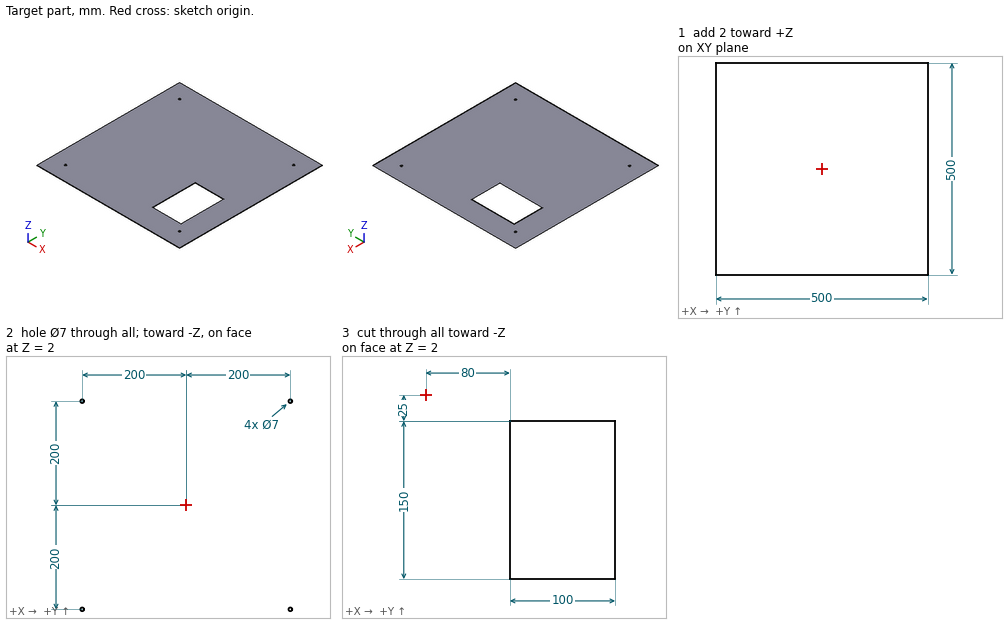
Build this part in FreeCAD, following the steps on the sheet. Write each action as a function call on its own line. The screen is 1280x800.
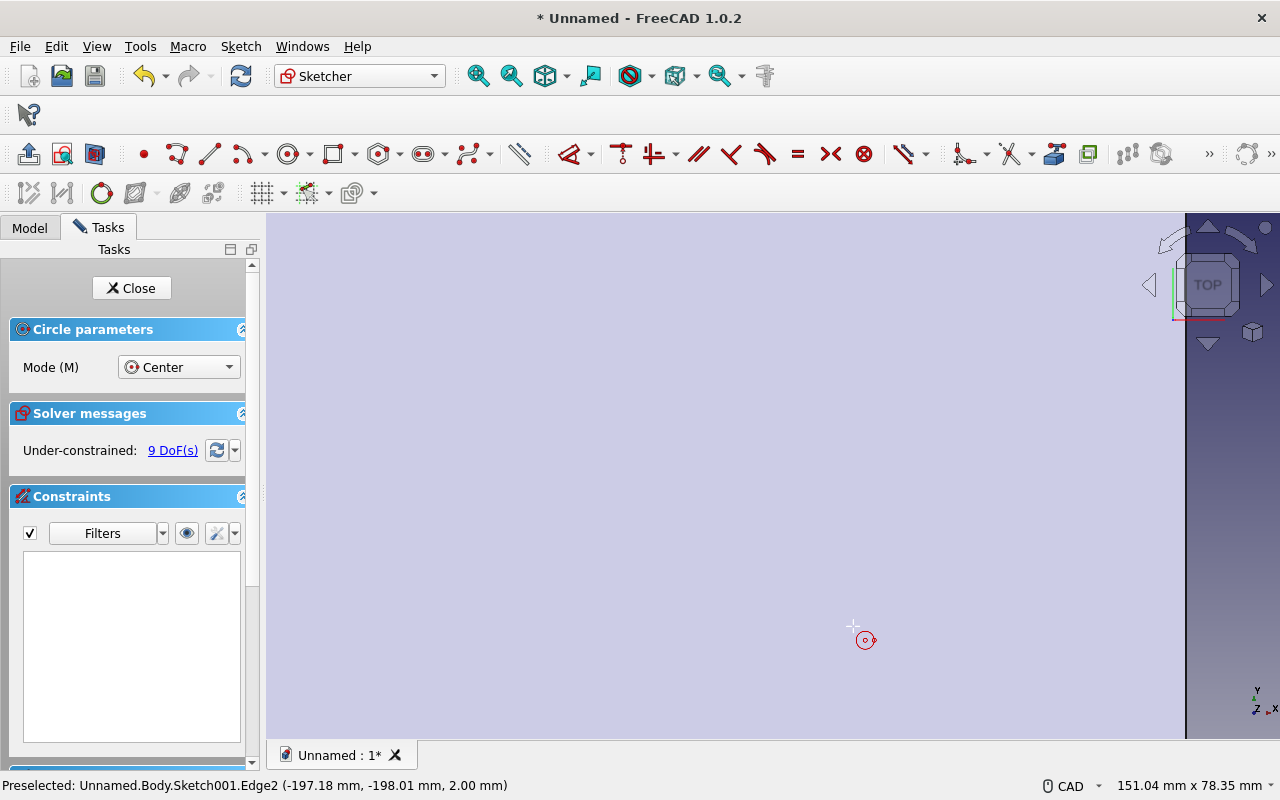
scroll(854, 626, down, 11)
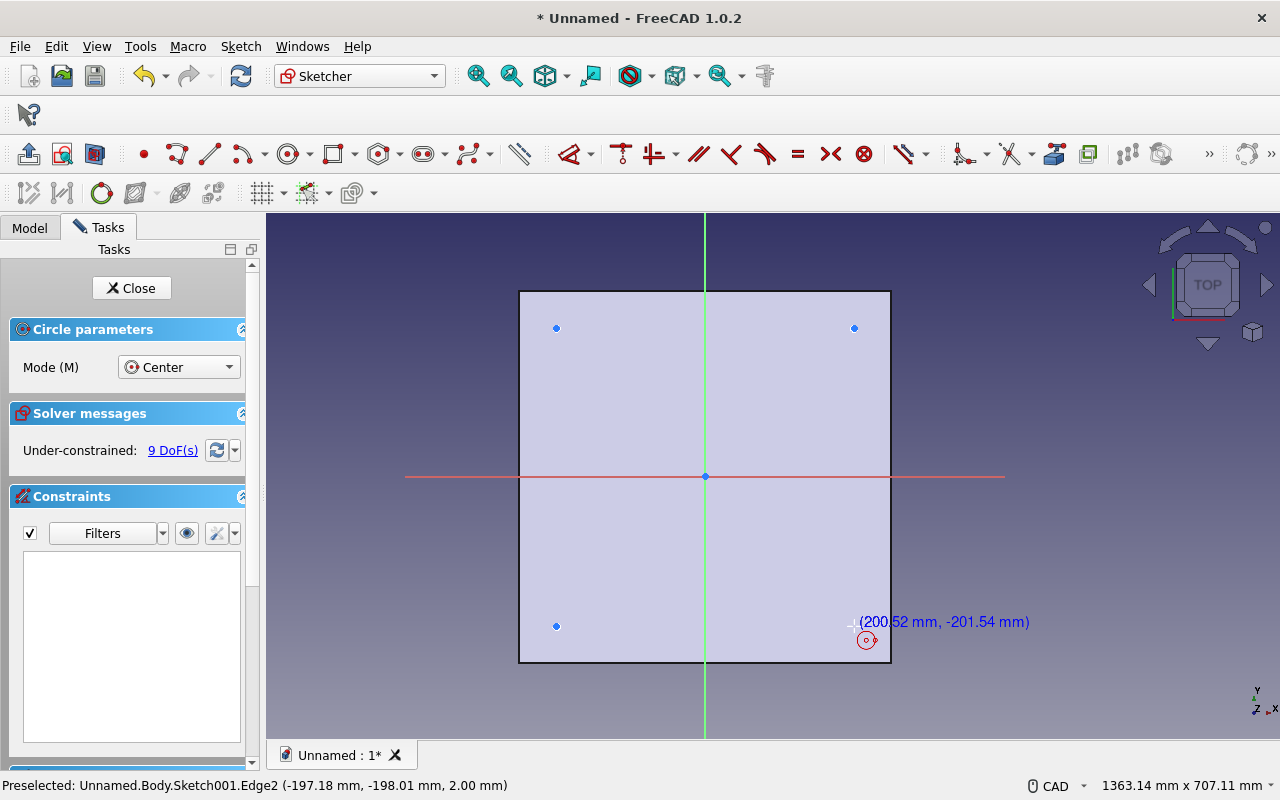
click(854, 626)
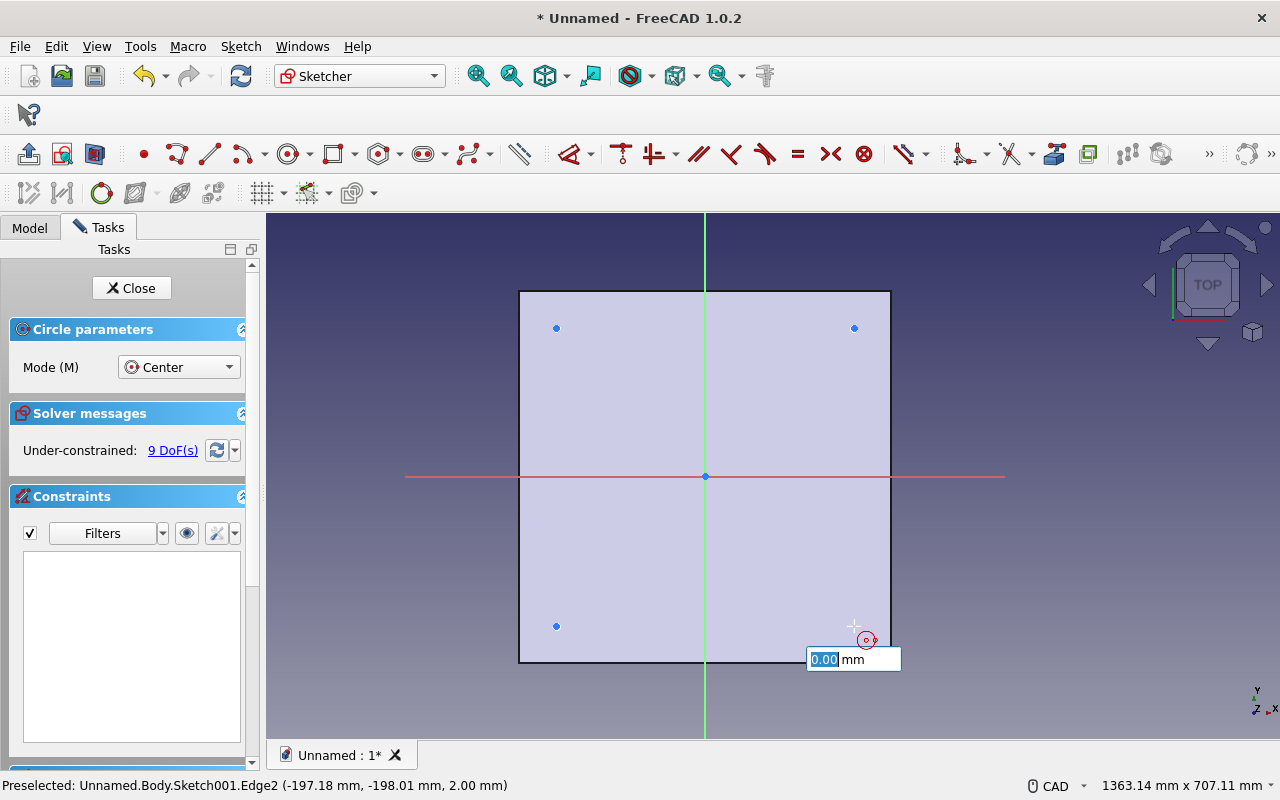
scroll(856, 624, up, 10)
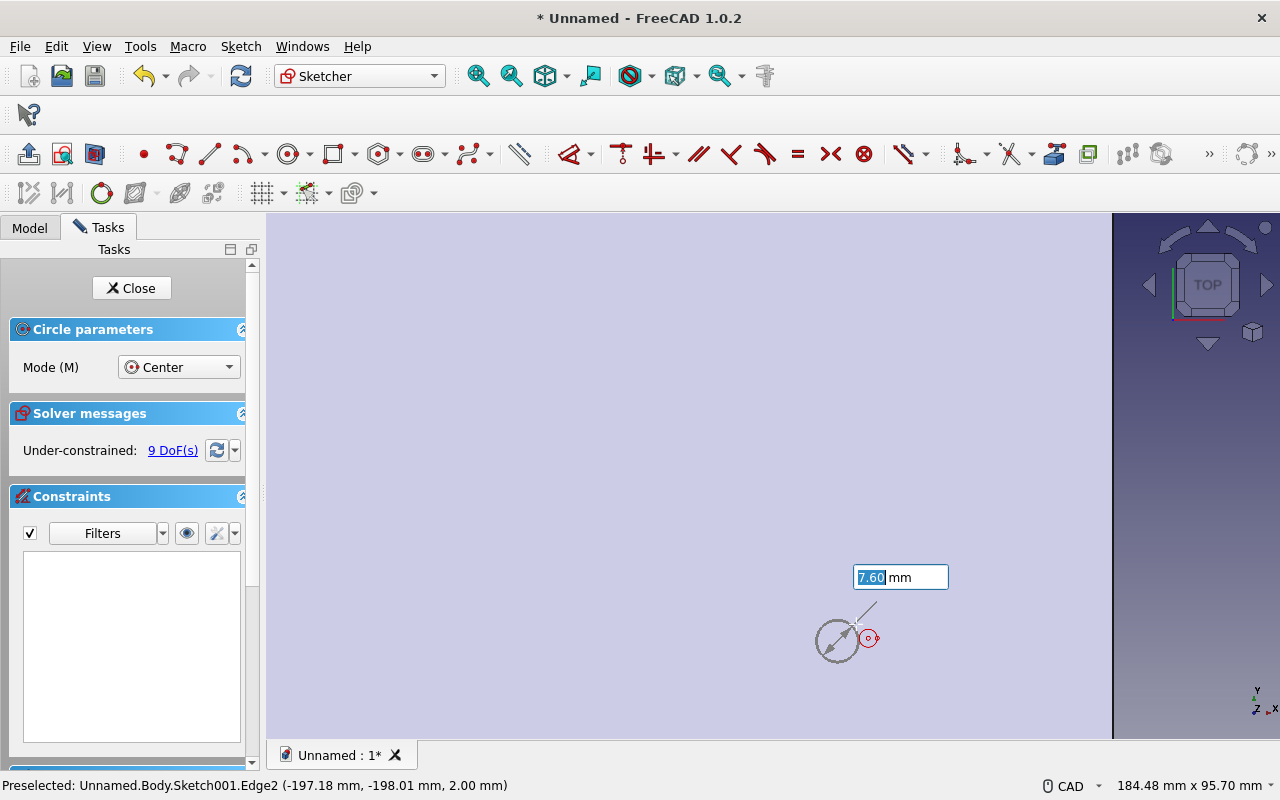
click(852, 618)
key(Escape)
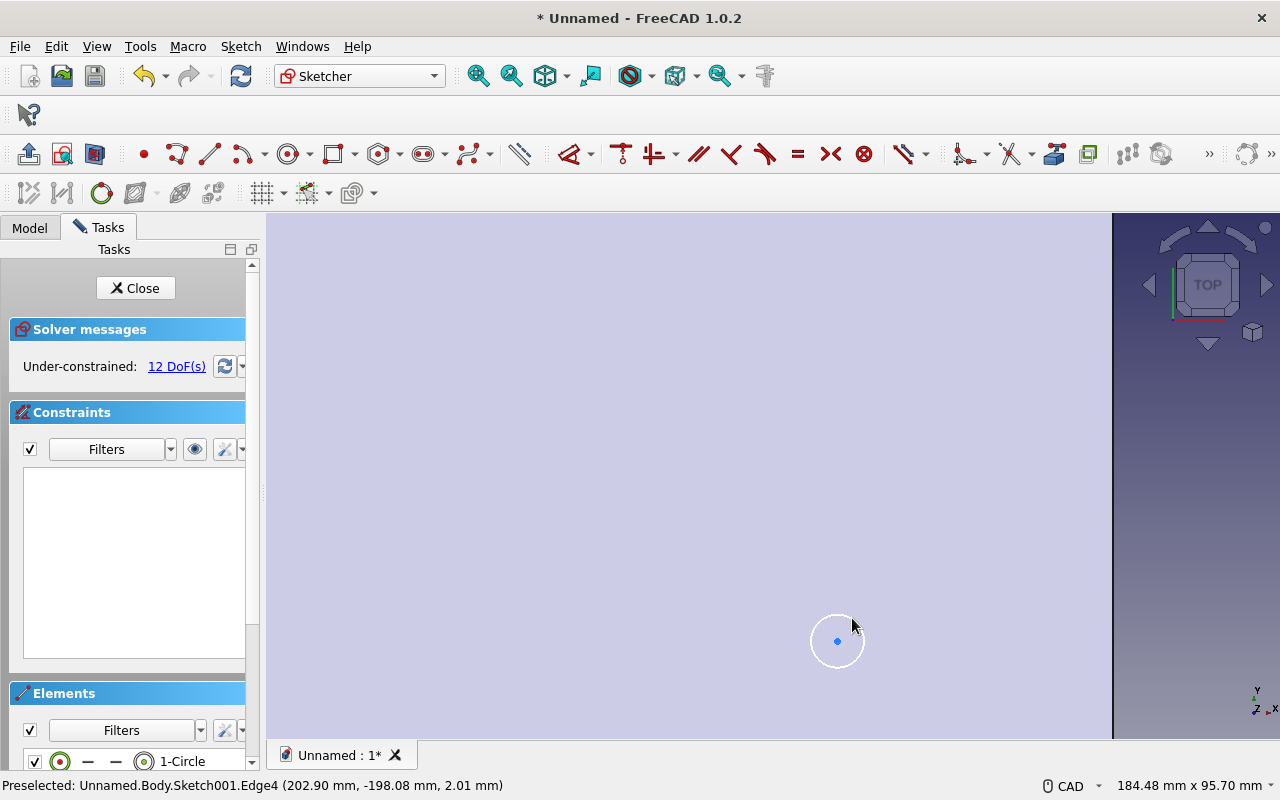
scroll(856, 624, down, 10)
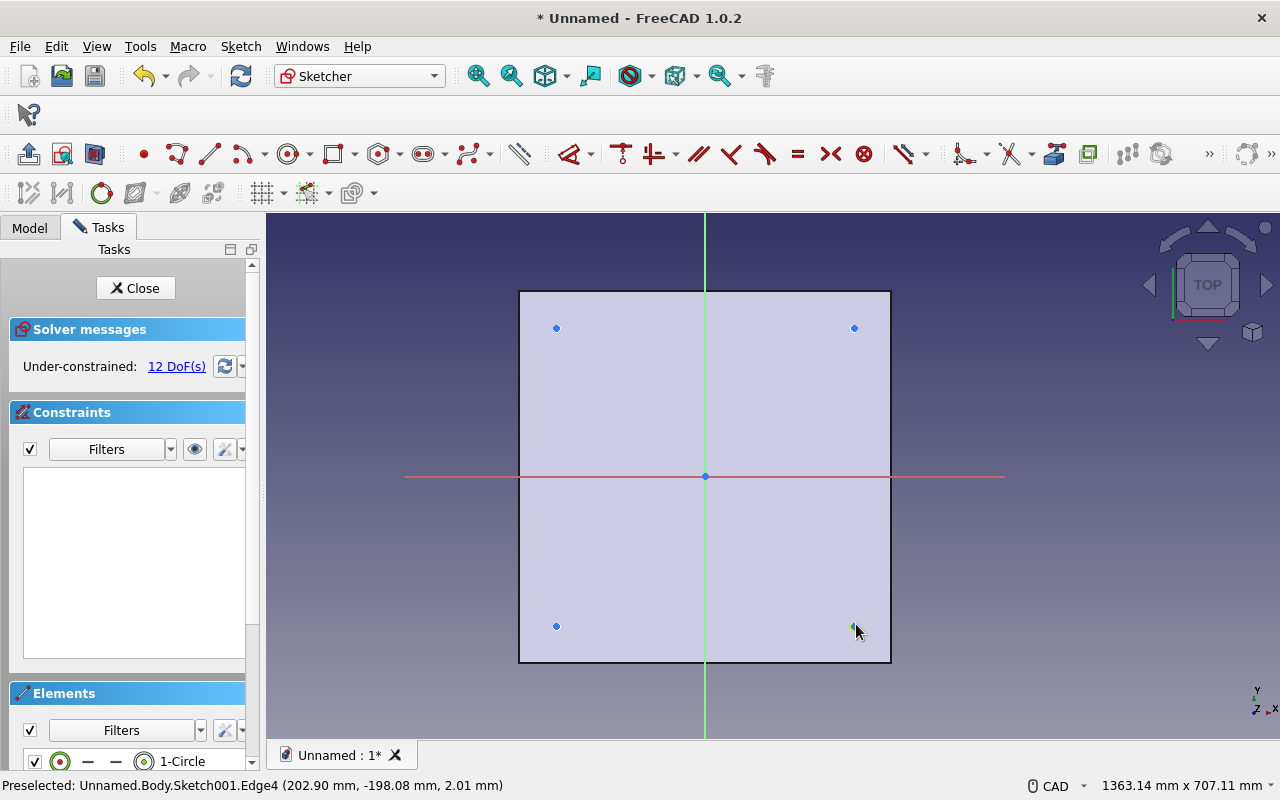
scroll(559, 327, up, 8)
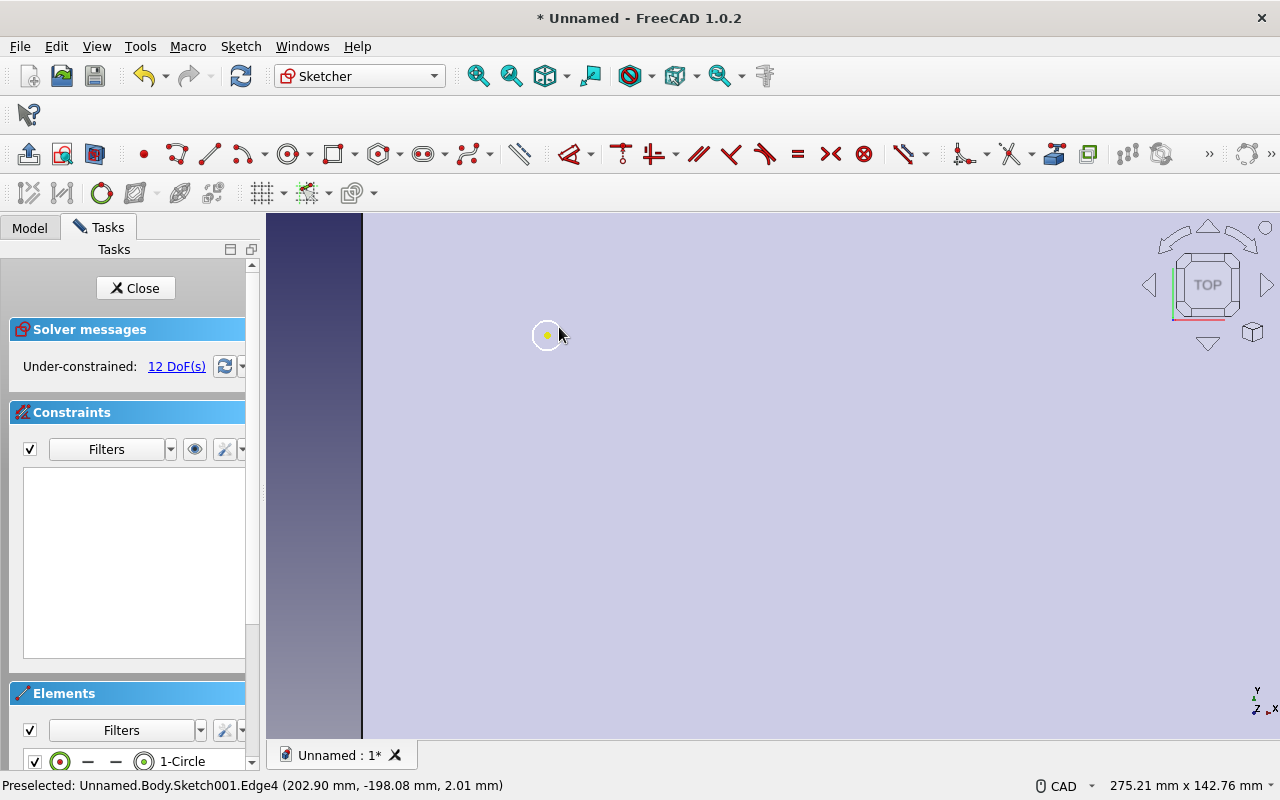
click(558, 325)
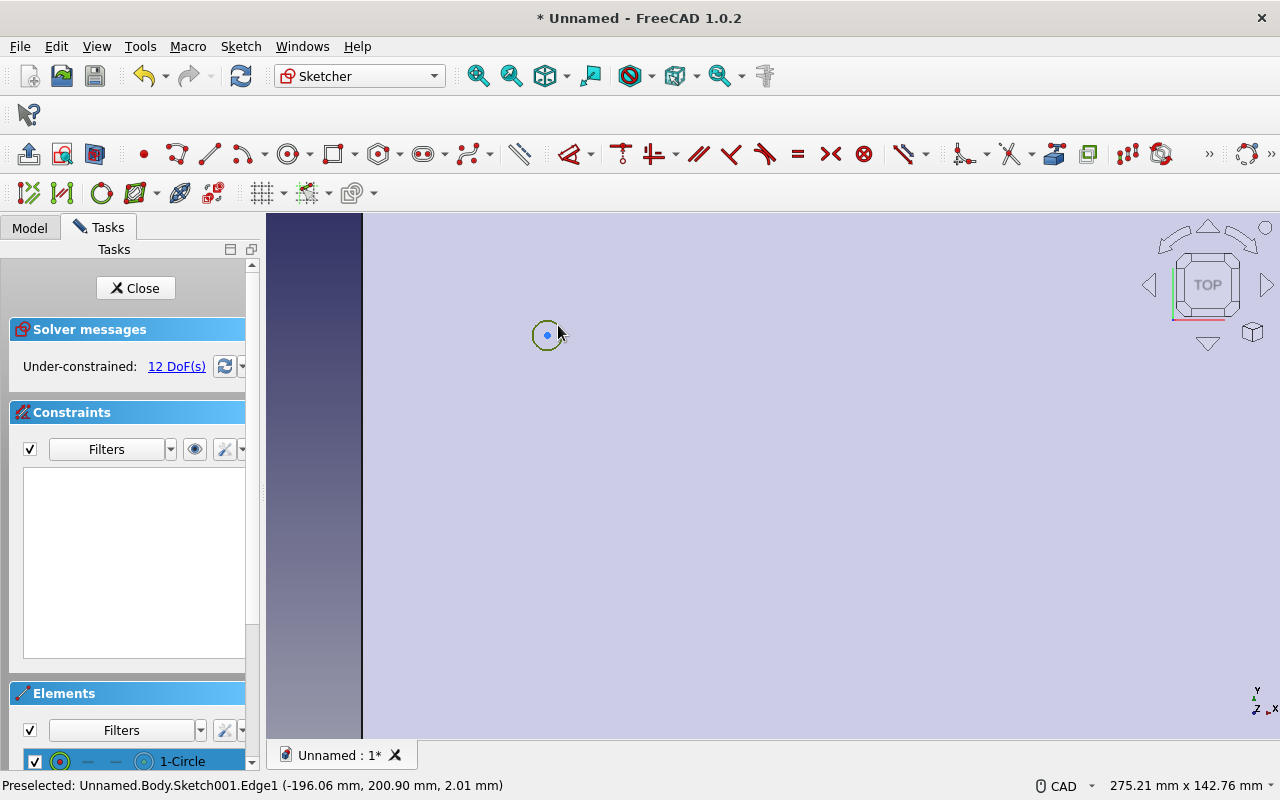
scroll(558, 326, down, 8)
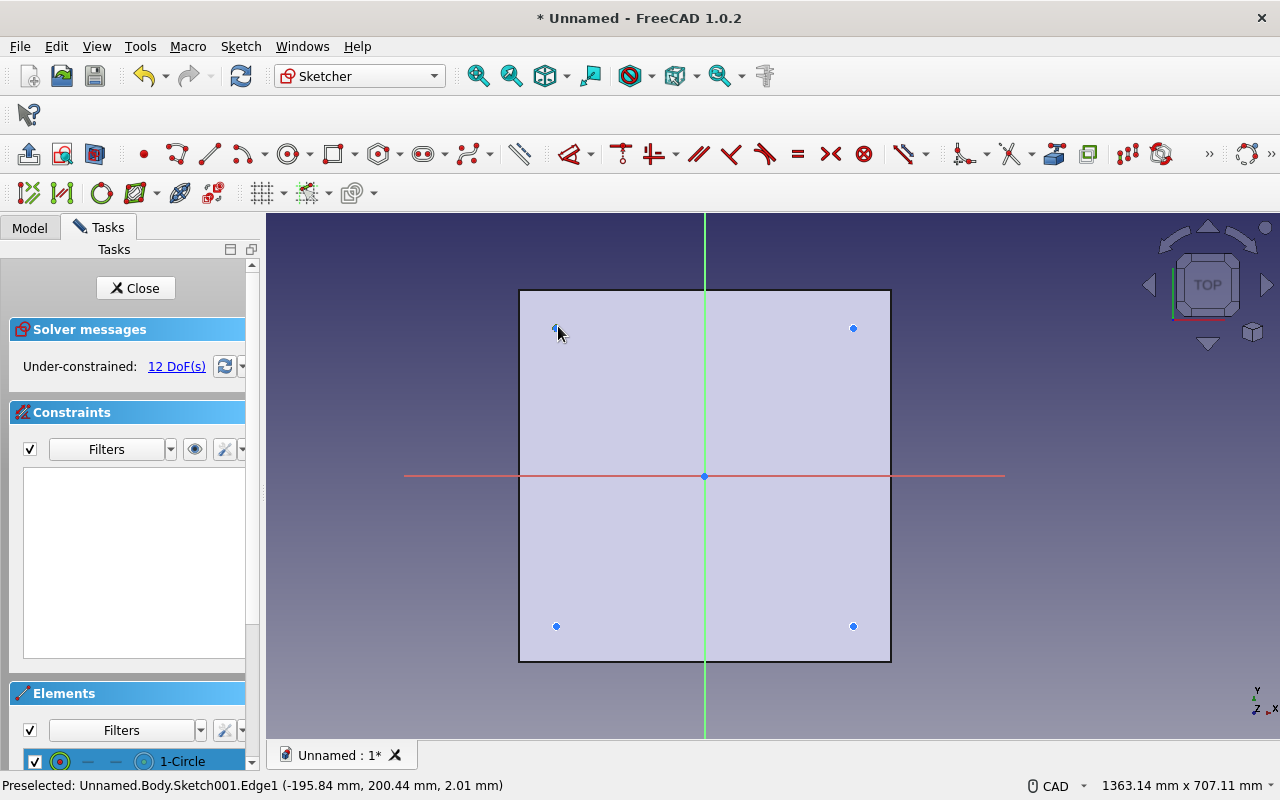
scroll(855, 326, up, 8)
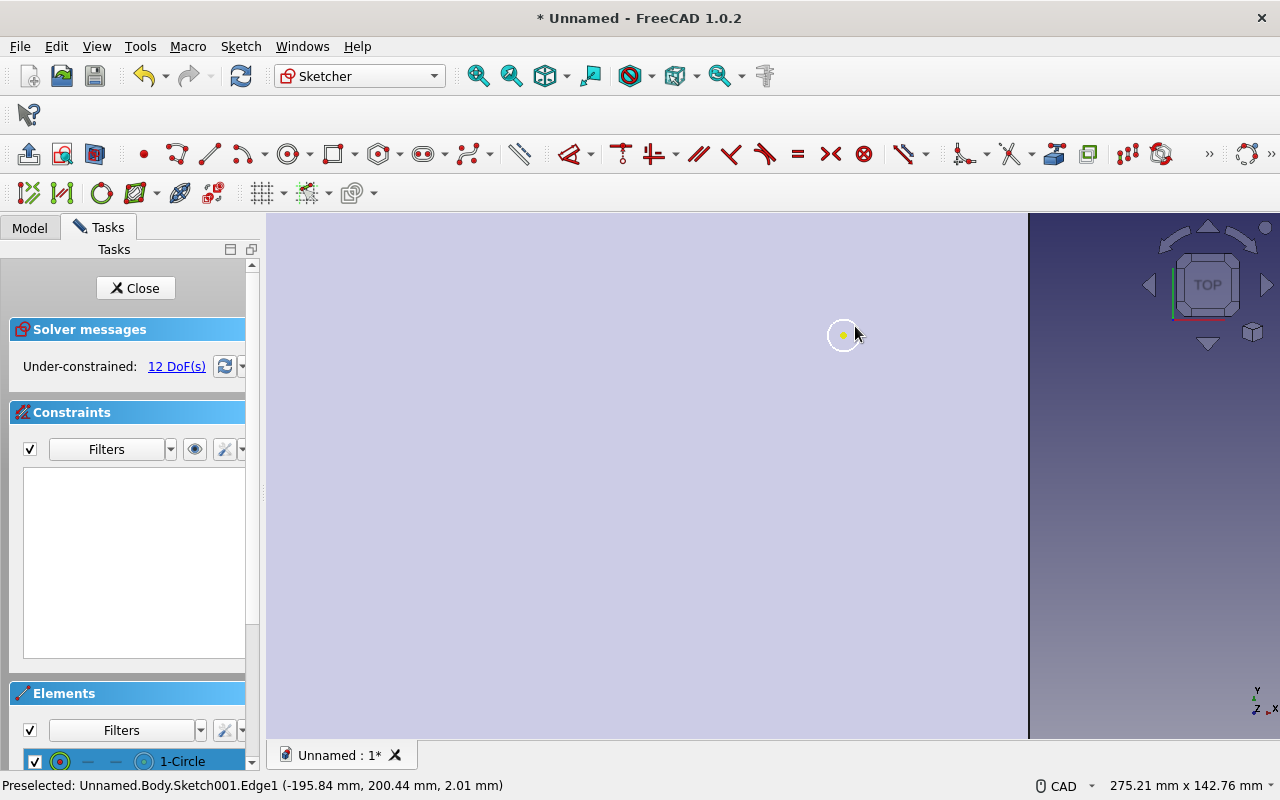
click(855, 324)